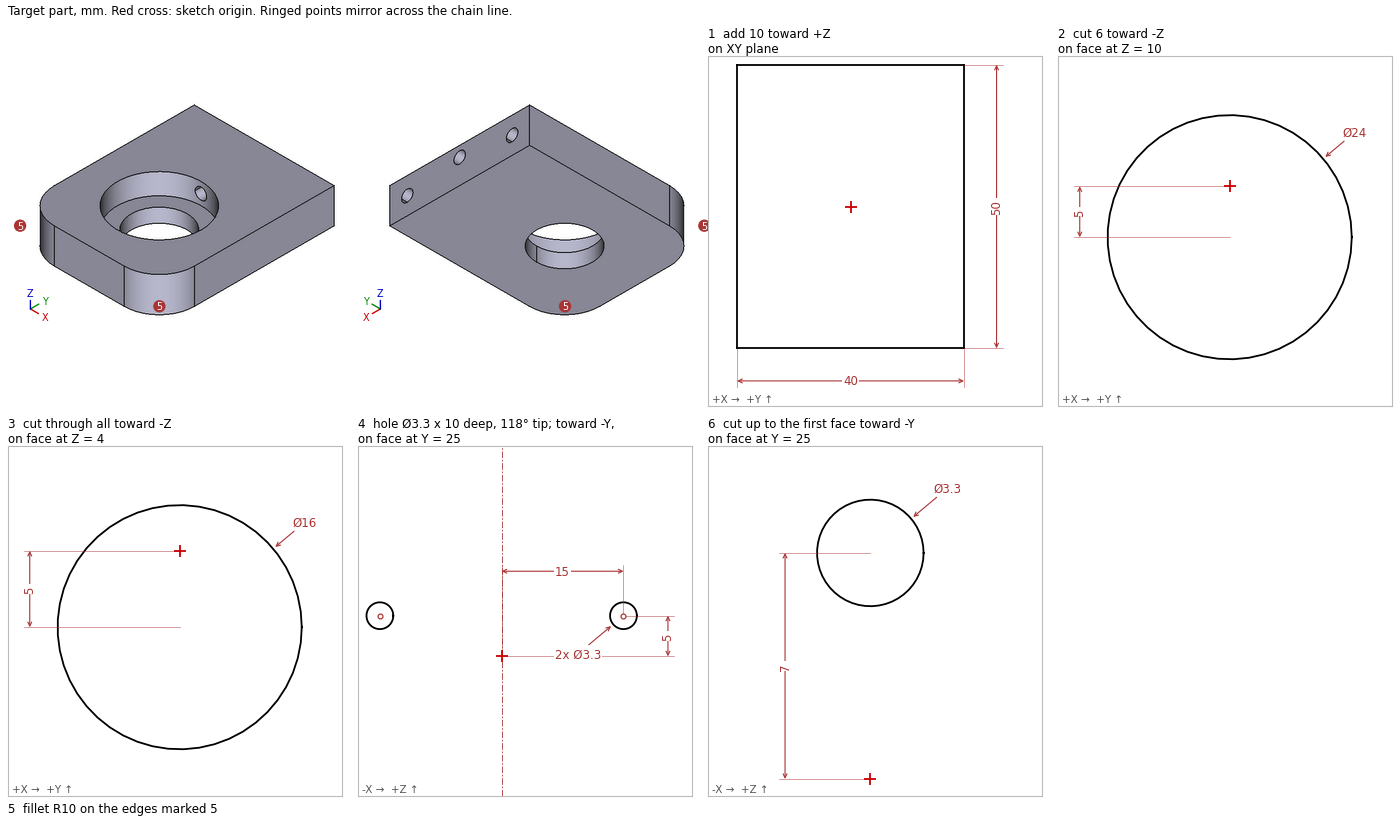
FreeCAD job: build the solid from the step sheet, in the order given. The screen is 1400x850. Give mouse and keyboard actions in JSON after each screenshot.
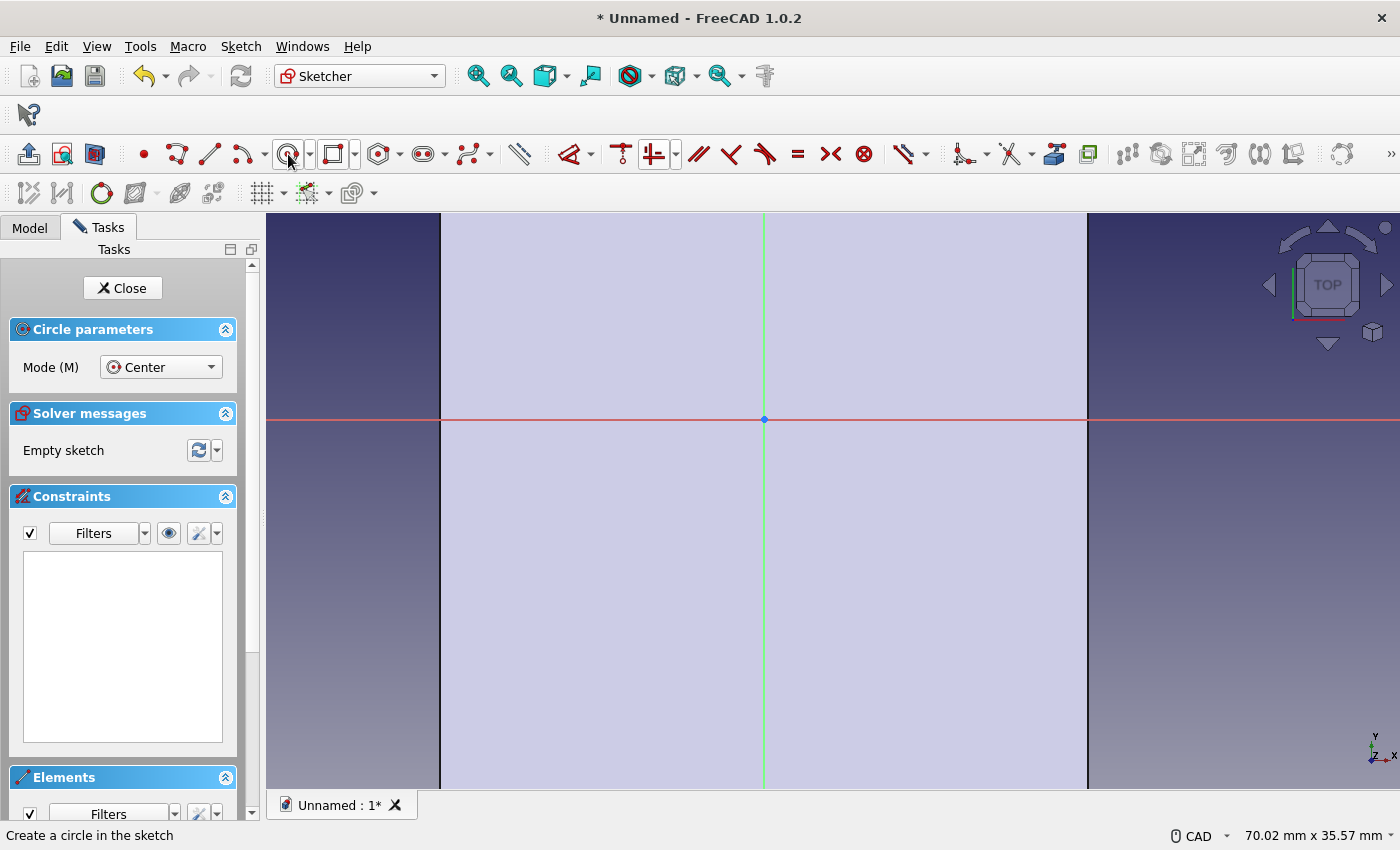
{"action": "left_click", "coordinate": [764, 501]}
{"action": "mouse_move", "coordinate": [902, 363]}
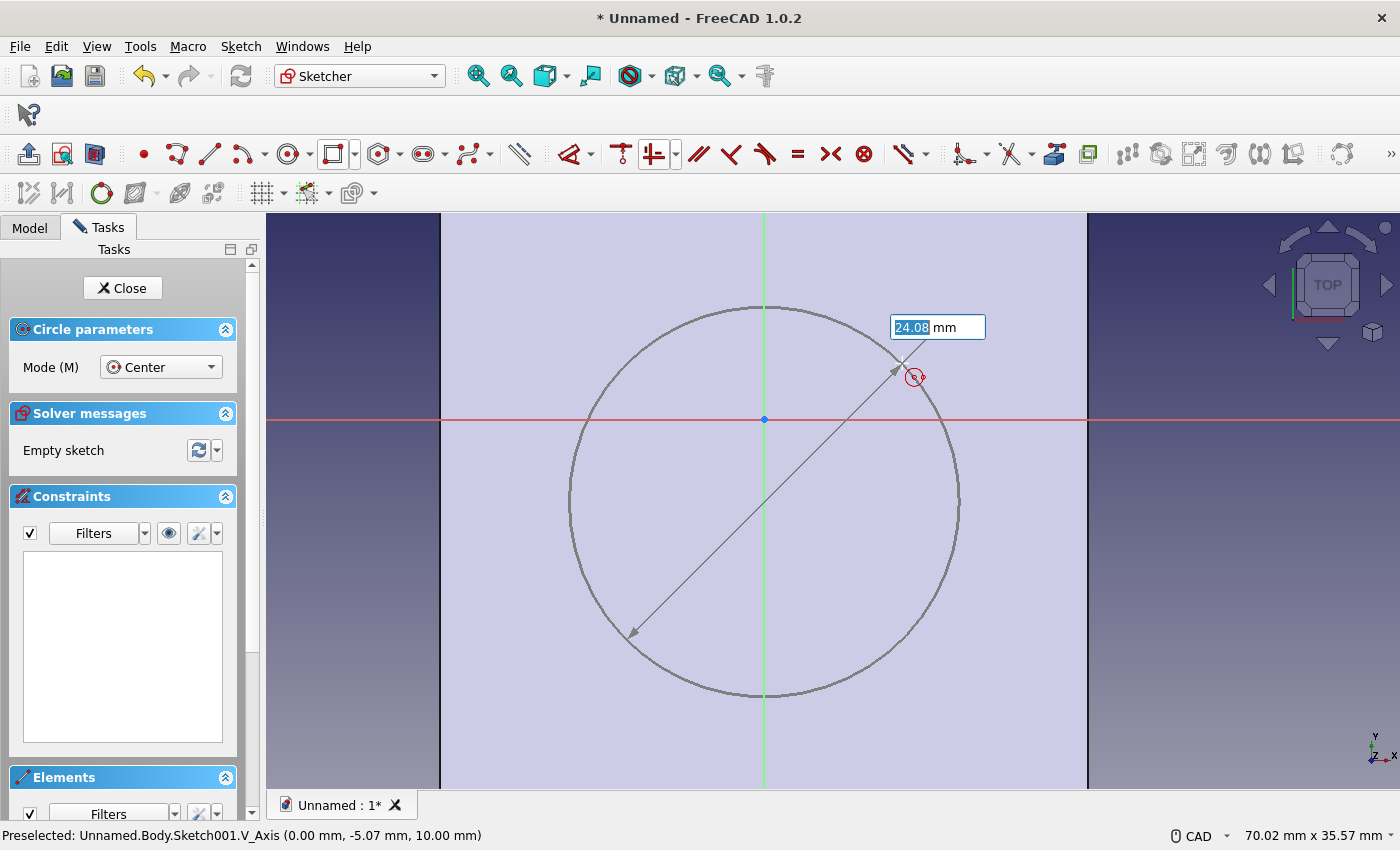
{"action": "type", "text": "24"}
{"action": "key", "text": "Return"}
{"action": "key", "text": "Escape"}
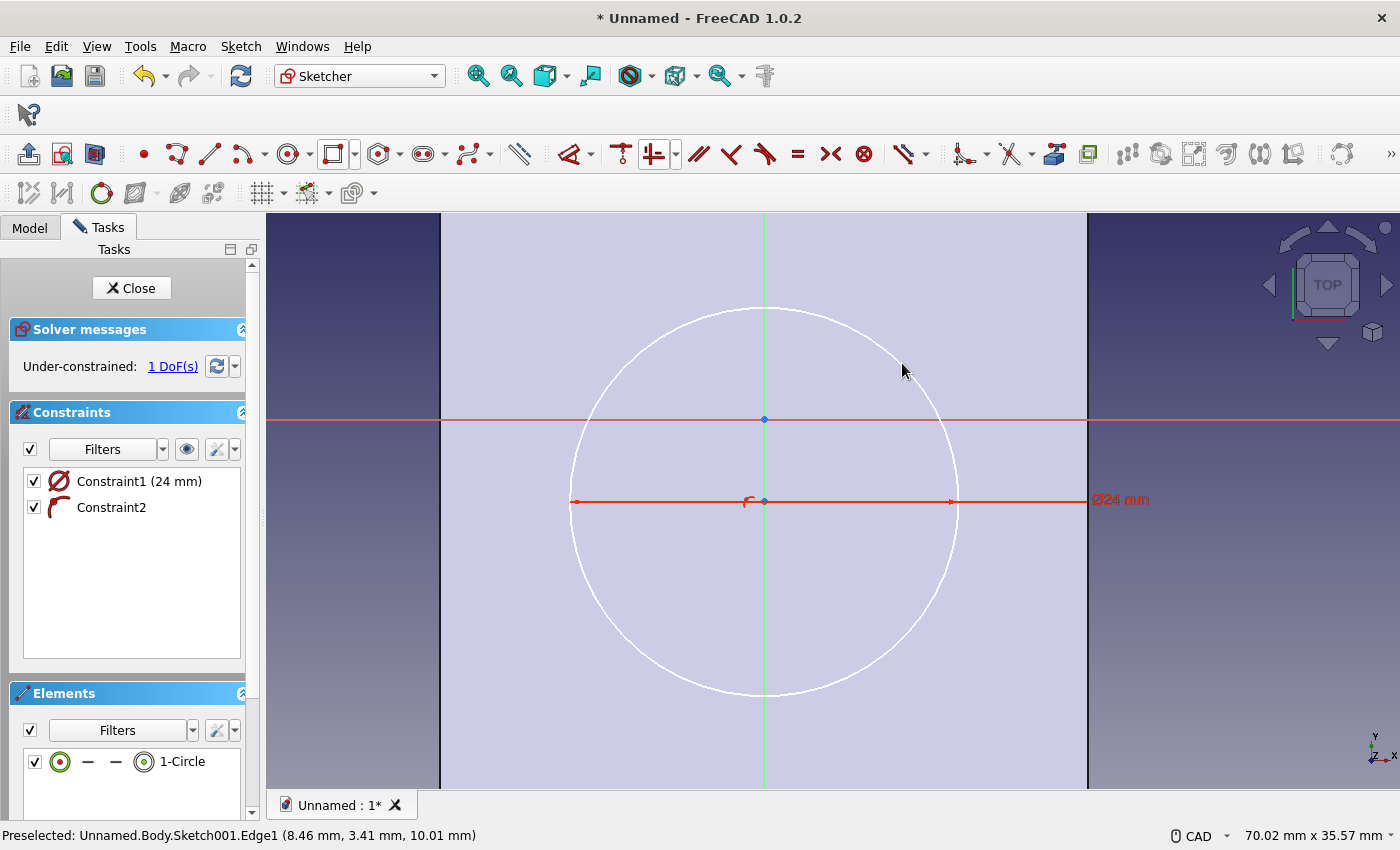
{"action": "left_click", "coordinate": [568, 154]}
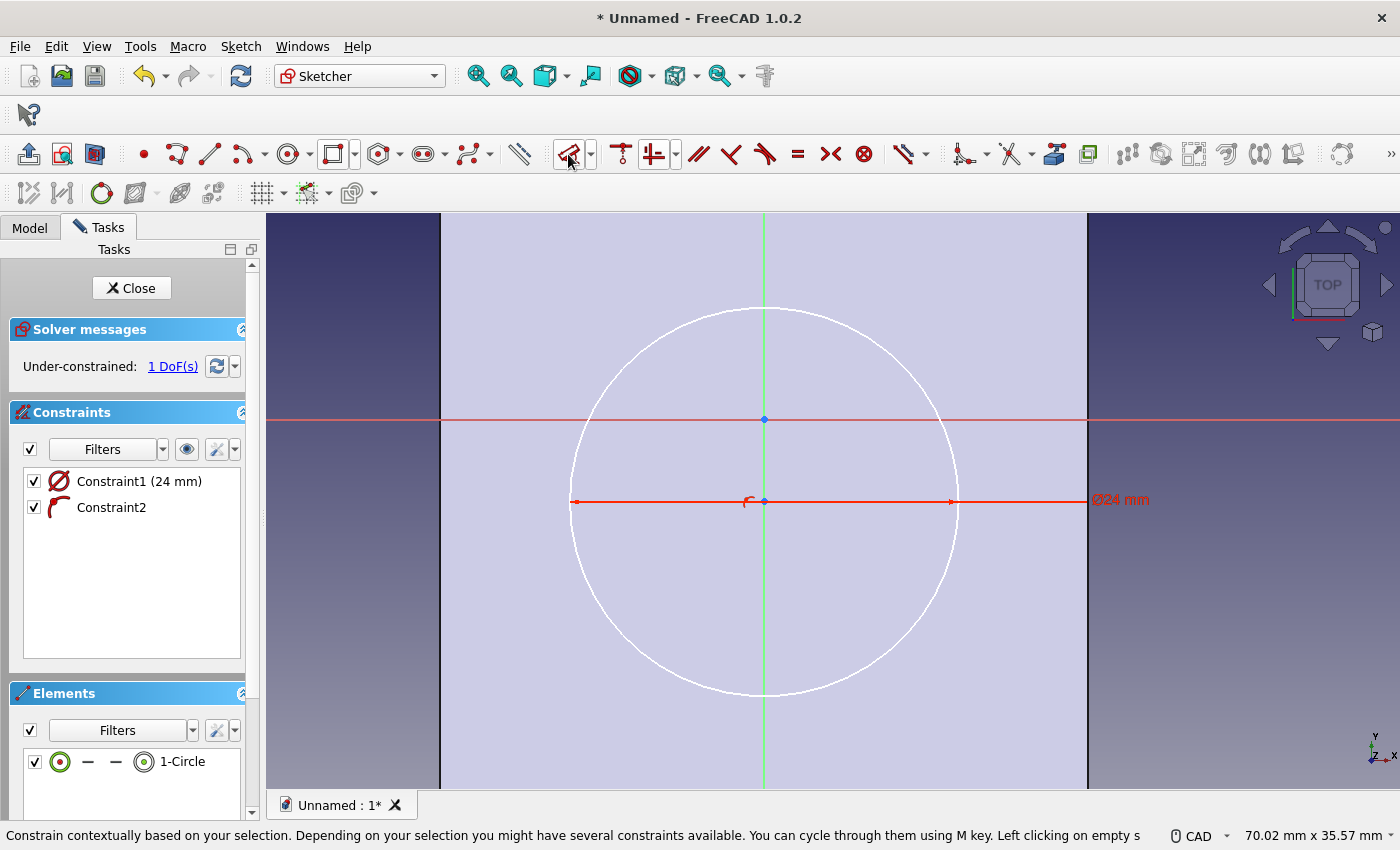
{"action": "left_click", "coordinate": [764, 502]}
{"action": "left_click", "coordinate": [798, 461]}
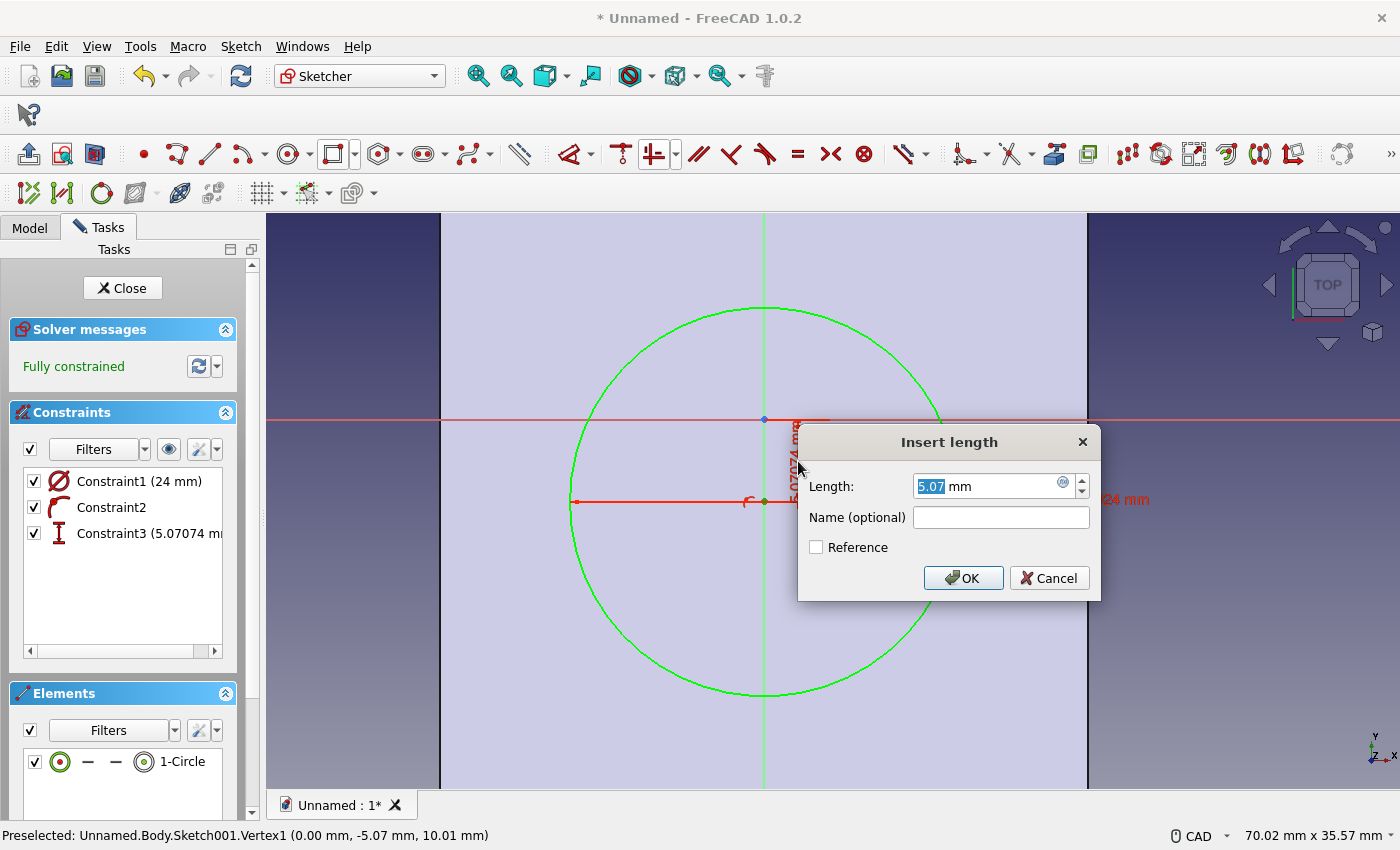
{"action": "type", "text": "5"}
{"action": "key", "text": "Return"}
{"action": "key", "text": "Escape"}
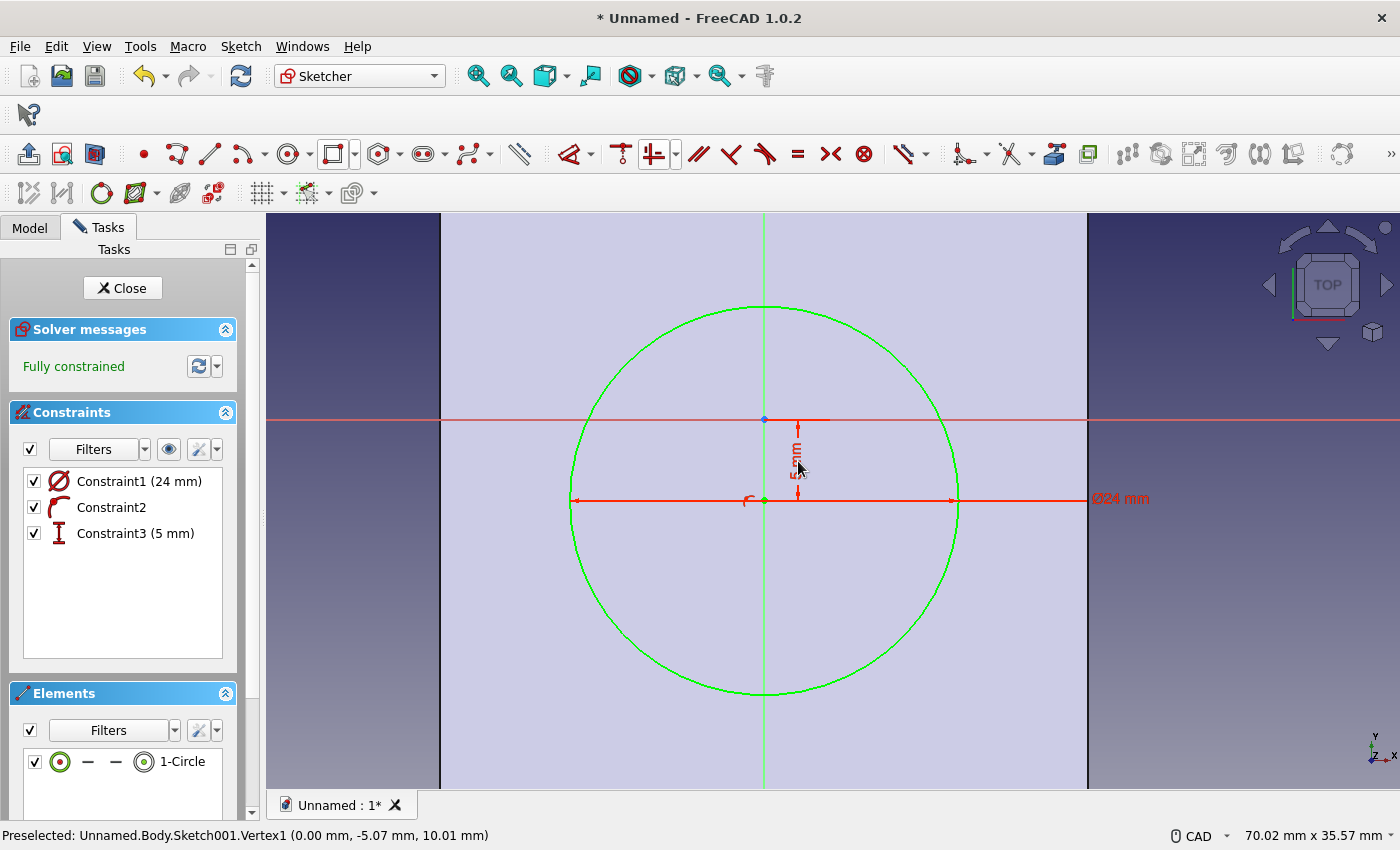
{"action": "left_click", "coordinate": [123, 288]}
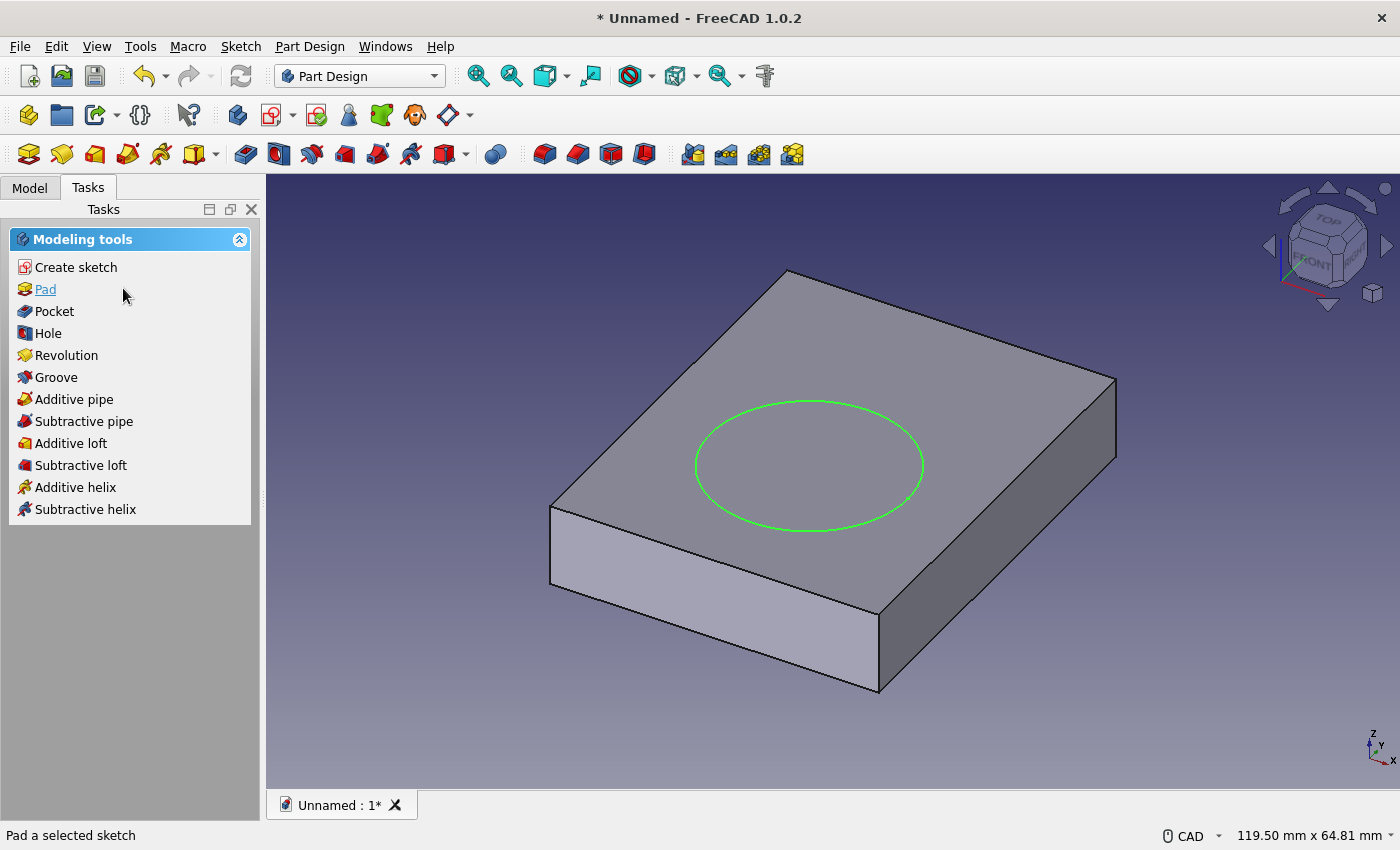
{"action": "left_click", "coordinate": [246, 154]}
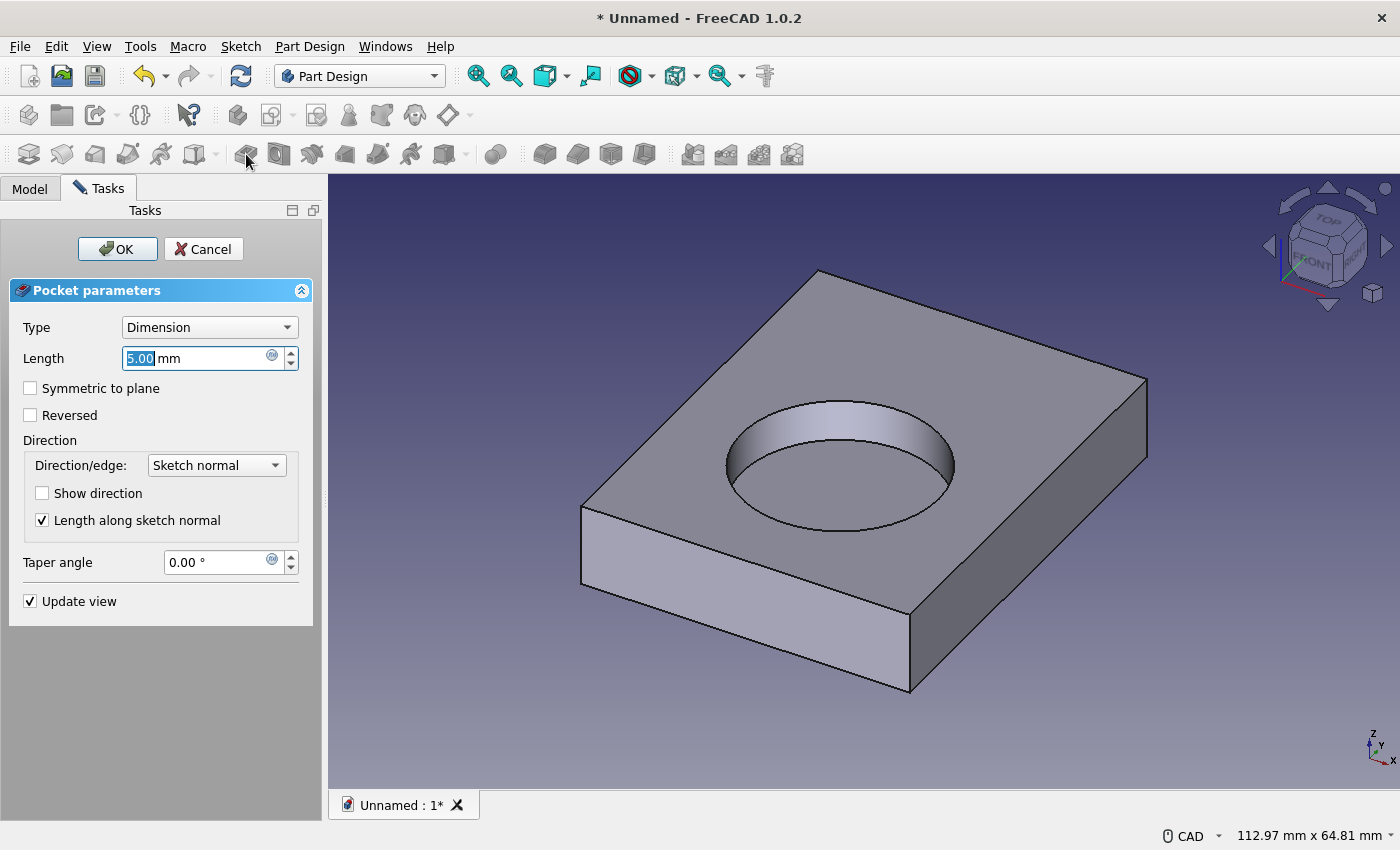
{"action": "type", "text": "6"}
{"action": "key", "text": "Tab"}